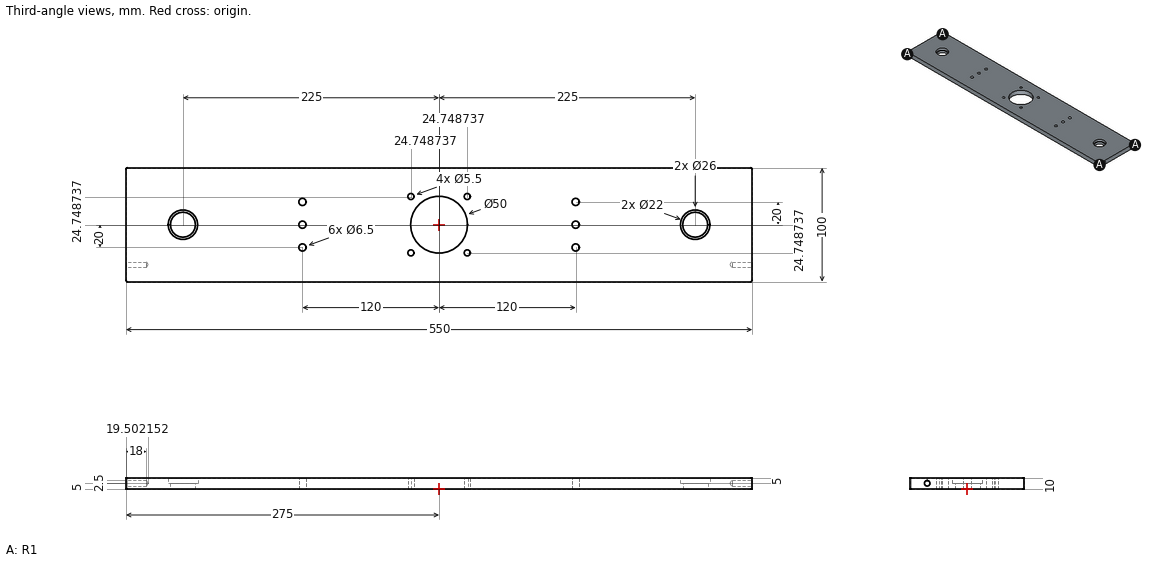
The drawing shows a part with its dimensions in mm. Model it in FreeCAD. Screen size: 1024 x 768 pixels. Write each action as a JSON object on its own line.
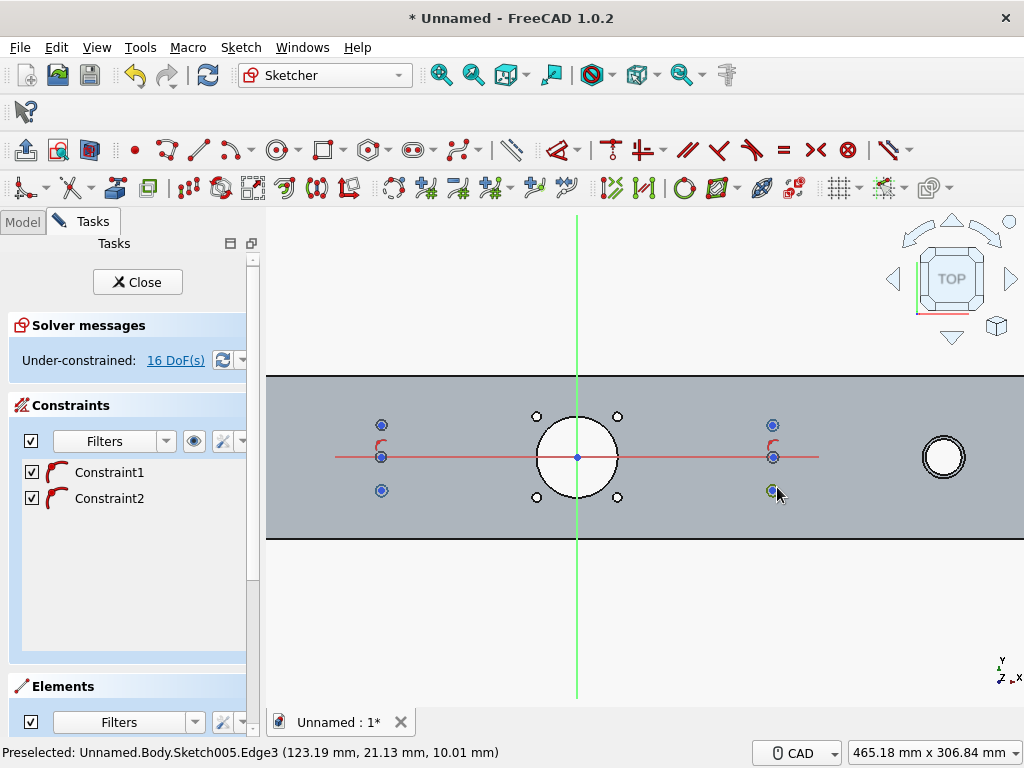
{"action": "scroll", "coordinate": [385, 421], "scroll_direction": "up", "scroll_amount": 5}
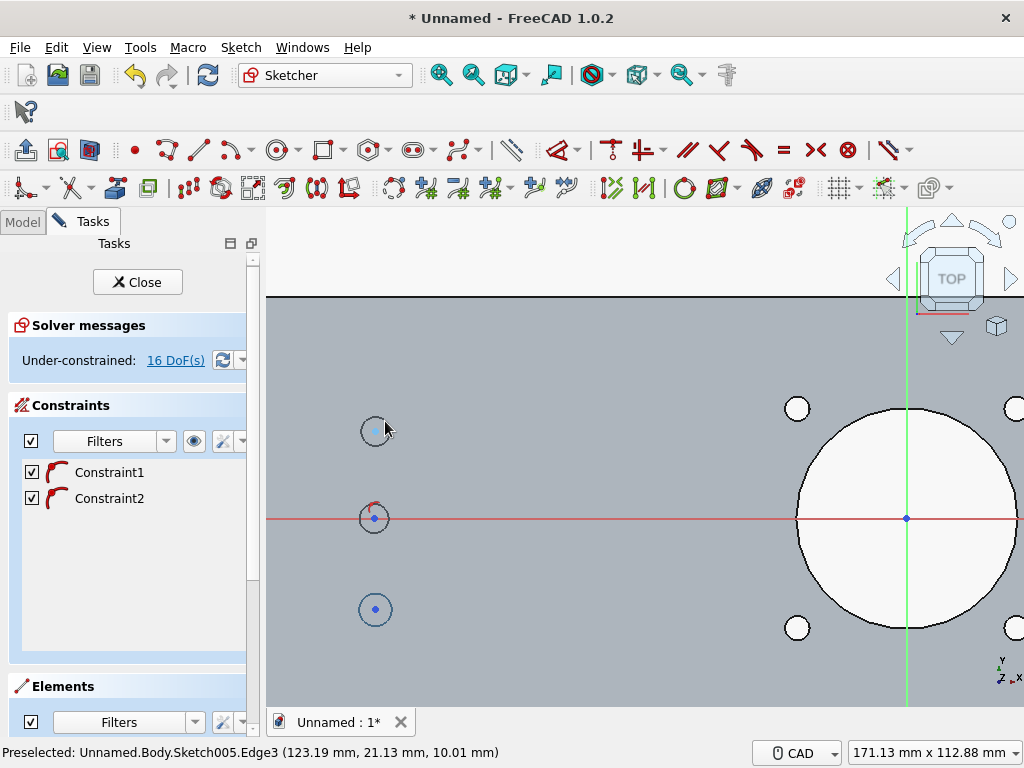
{"action": "left_click", "coordinate": [386, 421]}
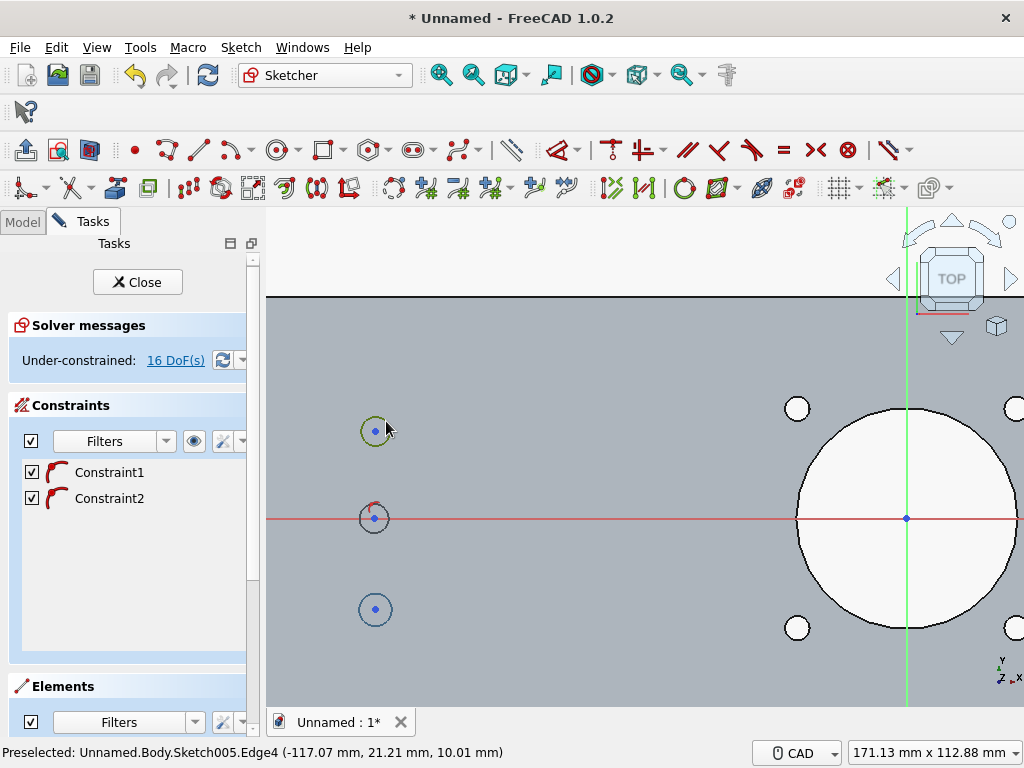
{"action": "scroll", "coordinate": [384, 508], "scroll_direction": "up", "scroll_amount": 2}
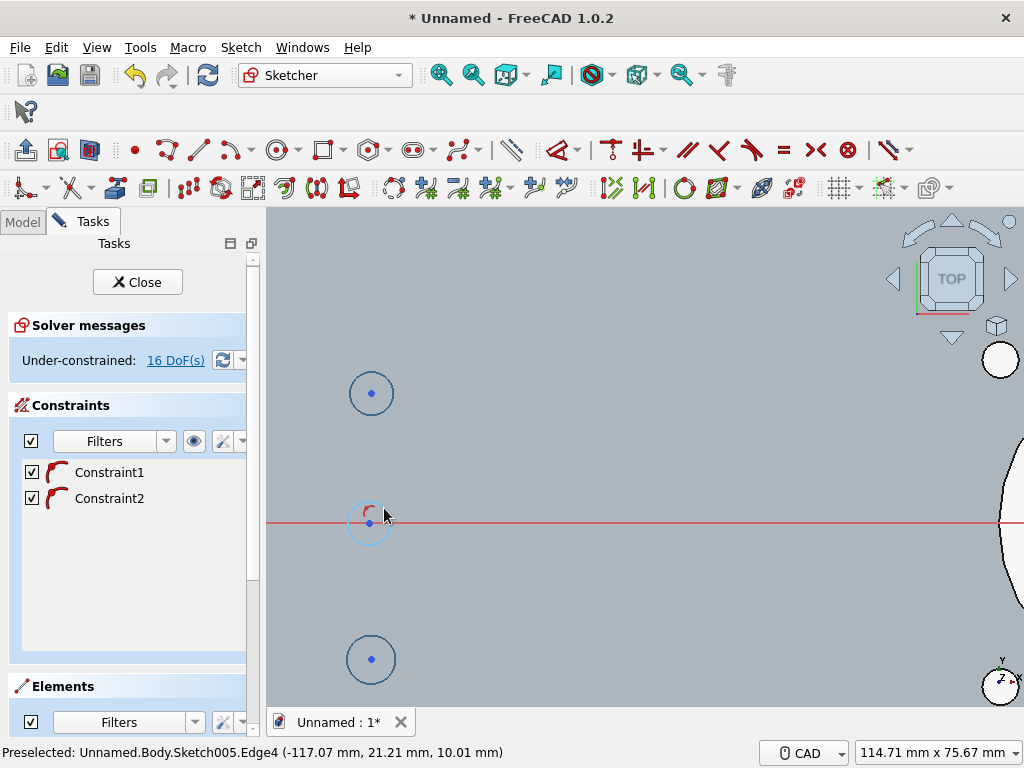
{"action": "left_click", "coordinate": [384, 508]}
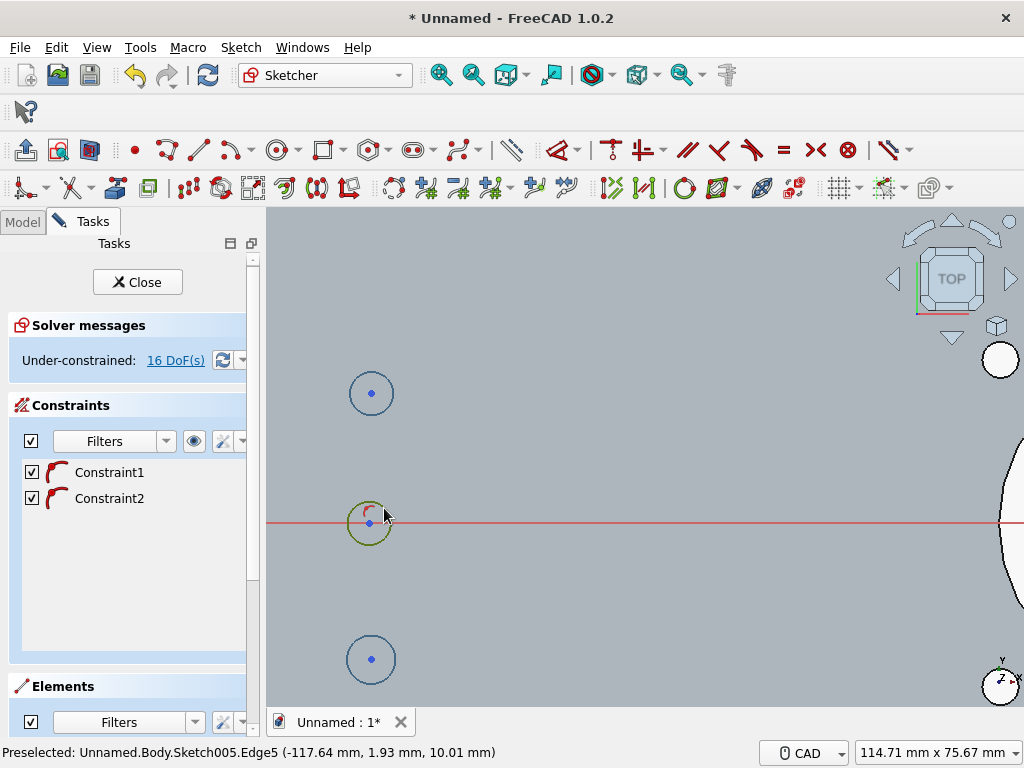
{"action": "scroll", "coordinate": [384, 435], "scroll_direction": "down", "scroll_amount": 7}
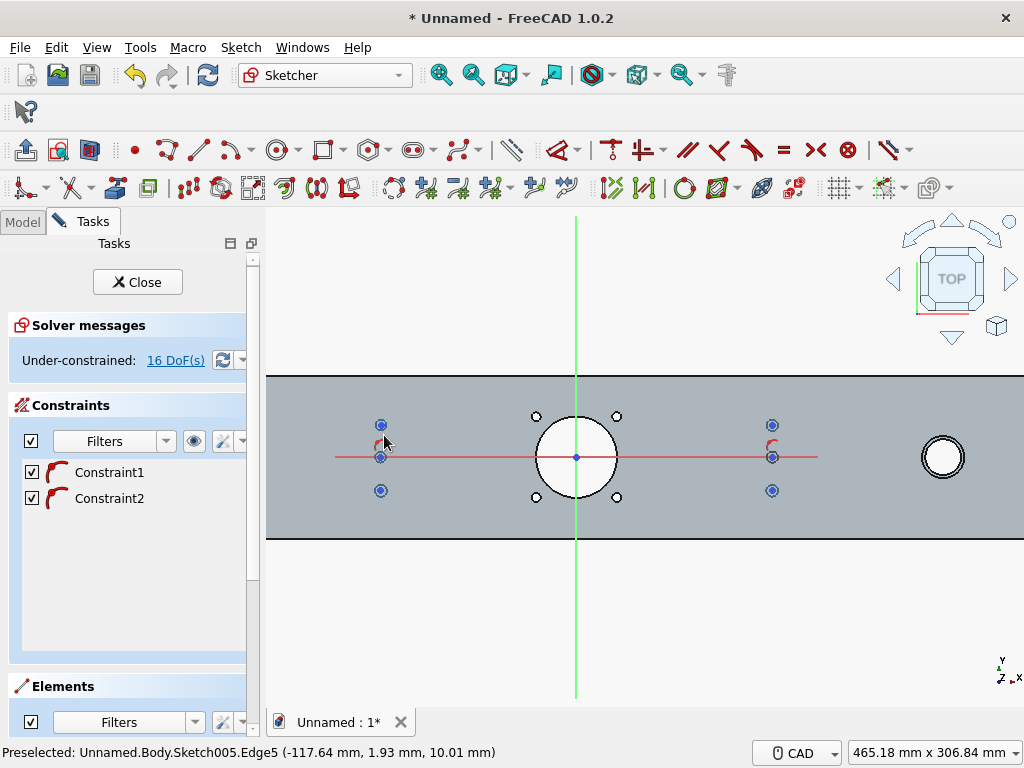
{"action": "scroll", "coordinate": [776, 453], "scroll_direction": "up", "scroll_amount": 7}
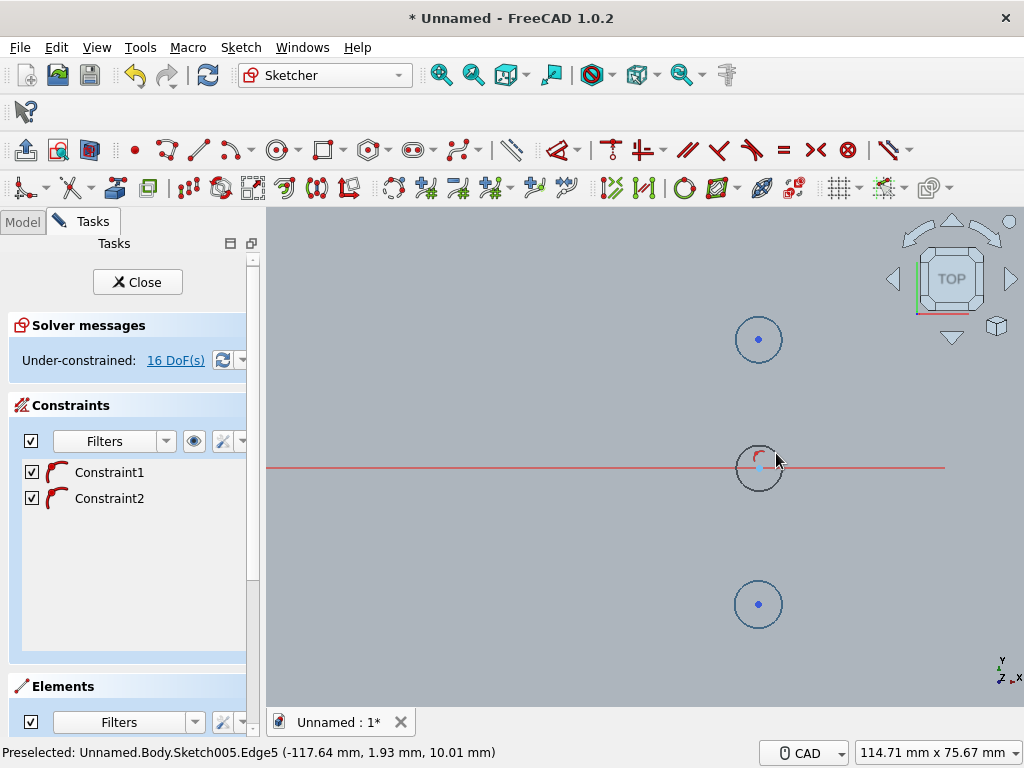
{"action": "left_click", "coordinate": [775, 452]}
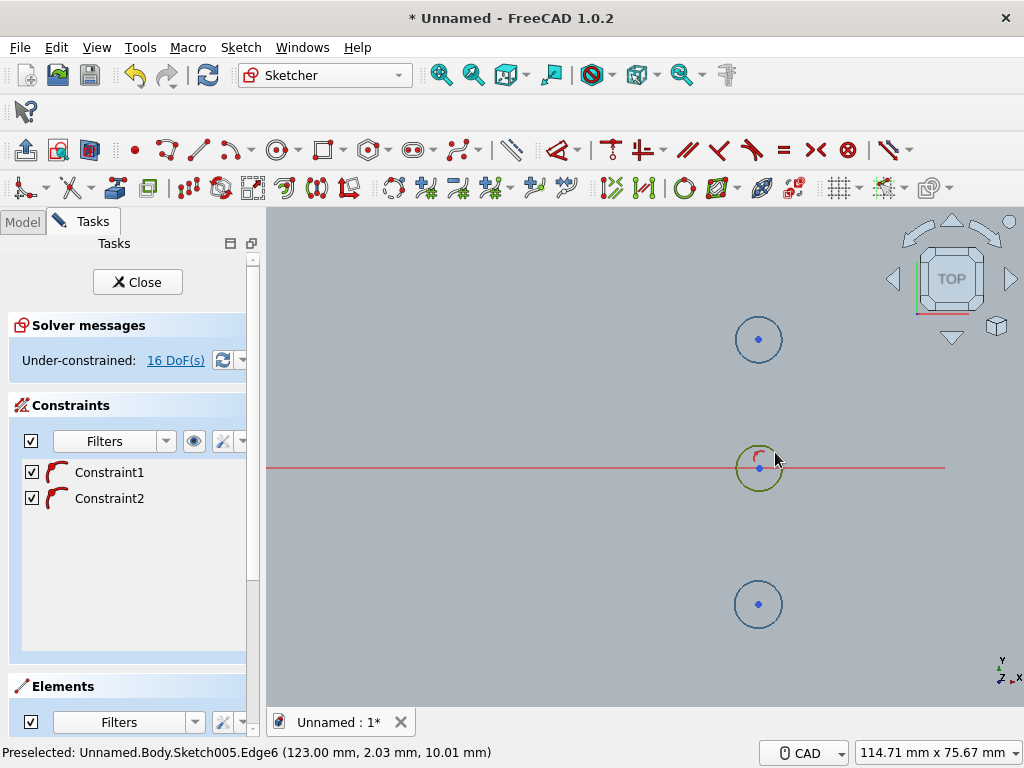
{"action": "key", "text": "e"}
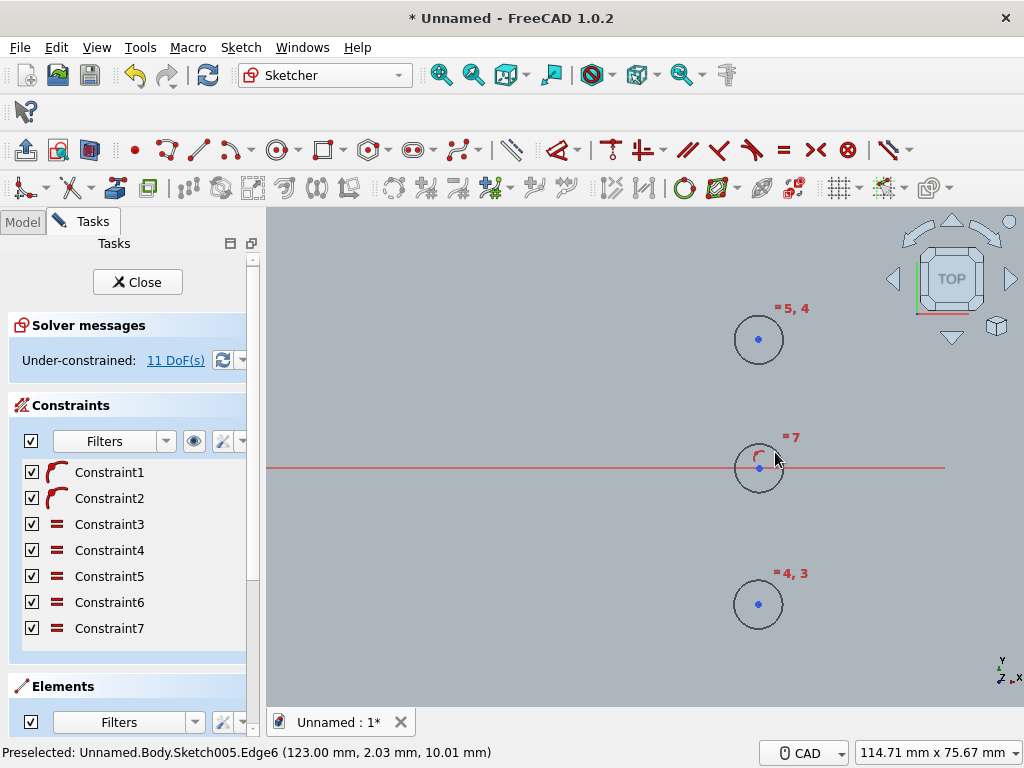
{"action": "scroll", "coordinate": [777, 453], "scroll_direction": "down", "scroll_amount": 7}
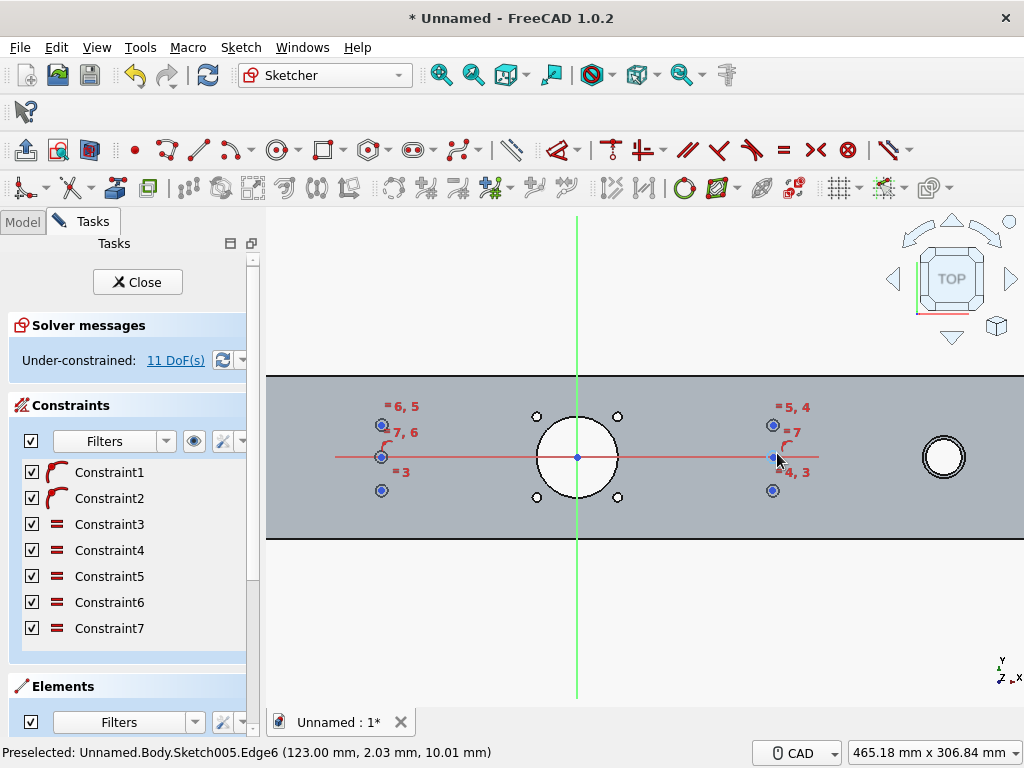
{"action": "left_click", "coordinate": [382, 491]}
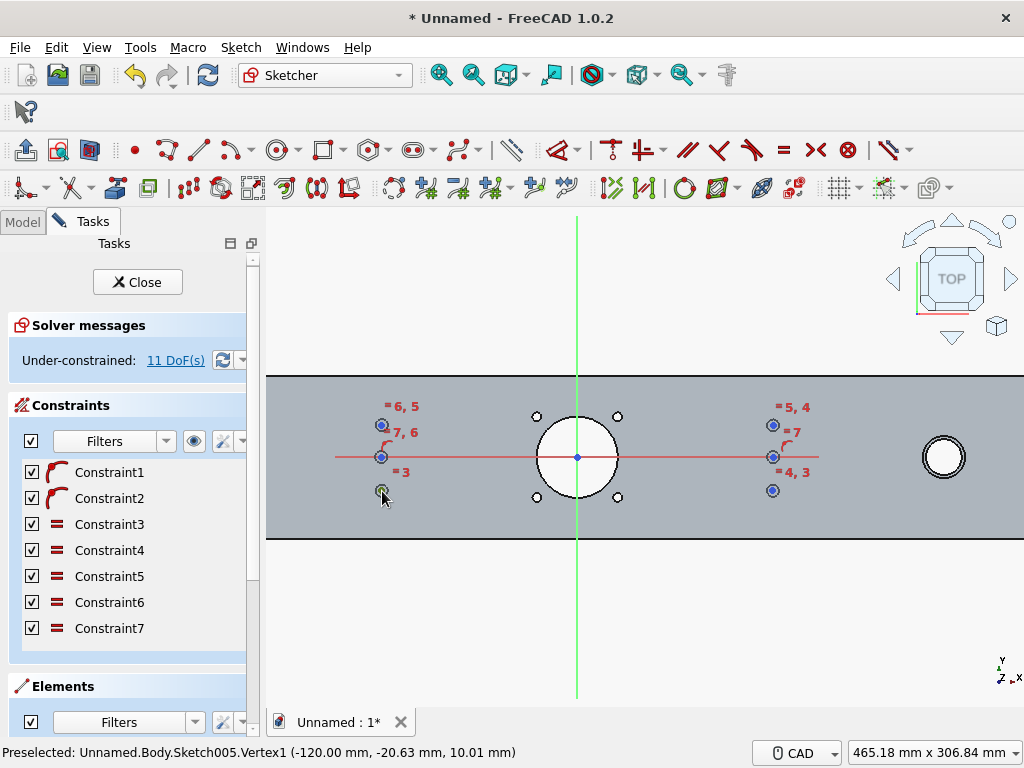
{"action": "left_click", "coordinate": [773, 491]}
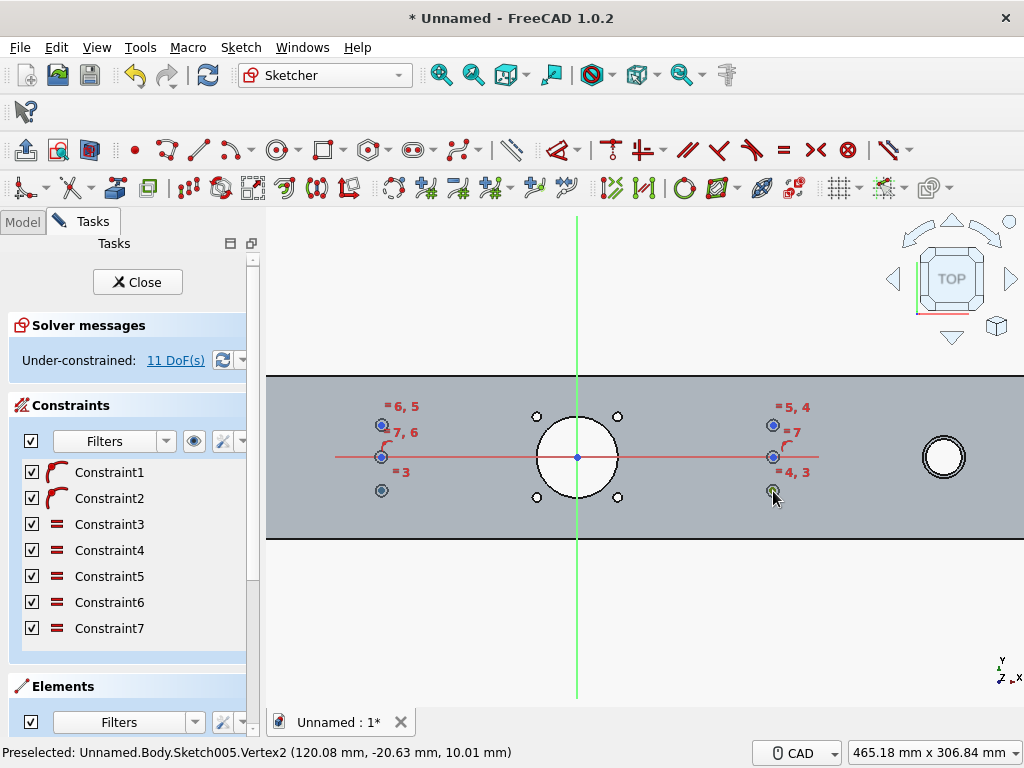
{"action": "key", "text": "h"}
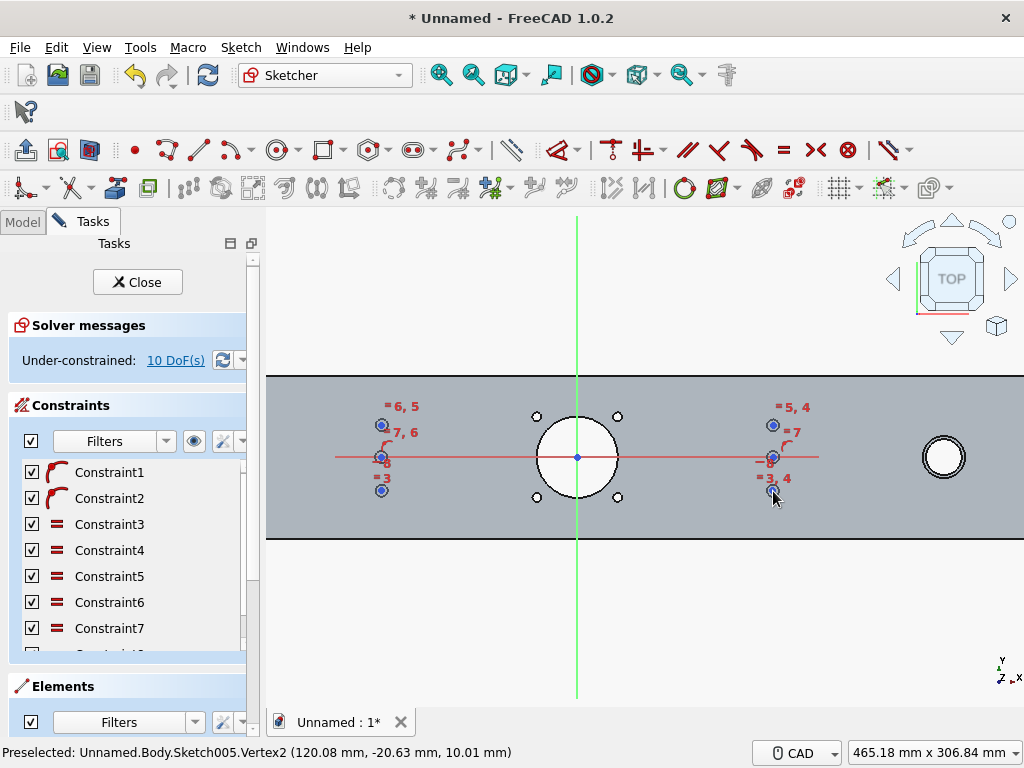
{"action": "left_click", "coordinate": [773, 491]}